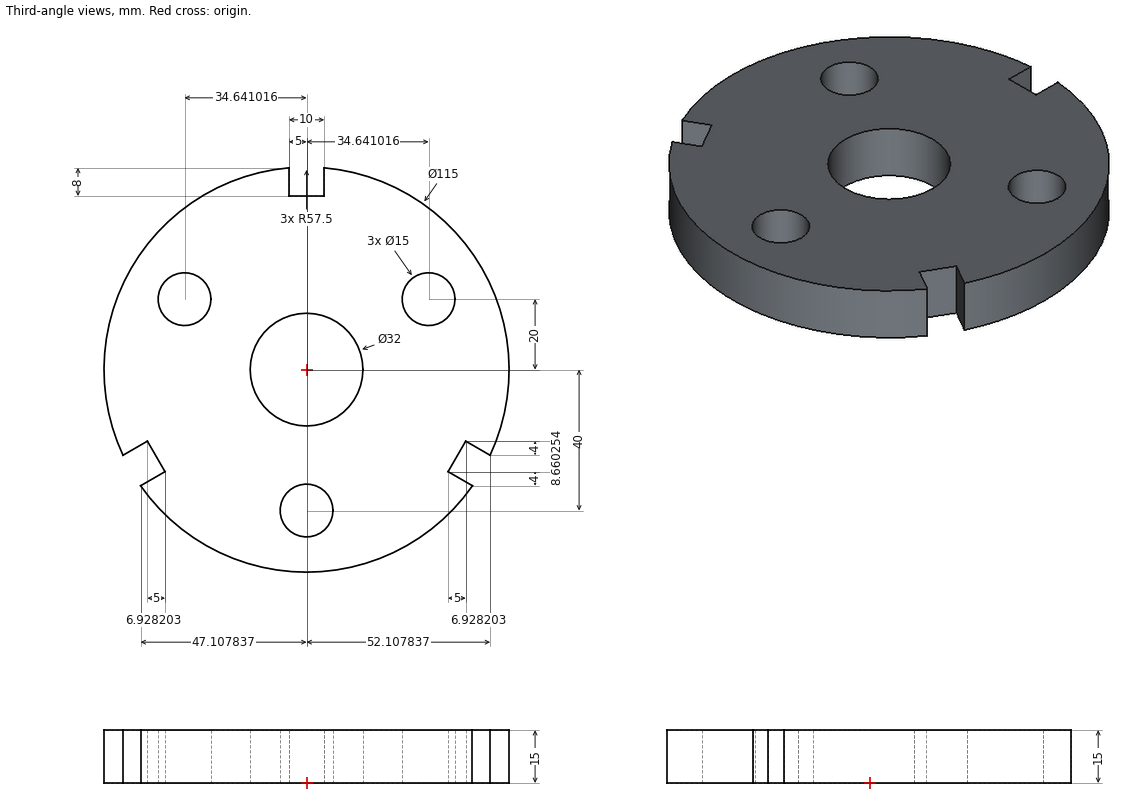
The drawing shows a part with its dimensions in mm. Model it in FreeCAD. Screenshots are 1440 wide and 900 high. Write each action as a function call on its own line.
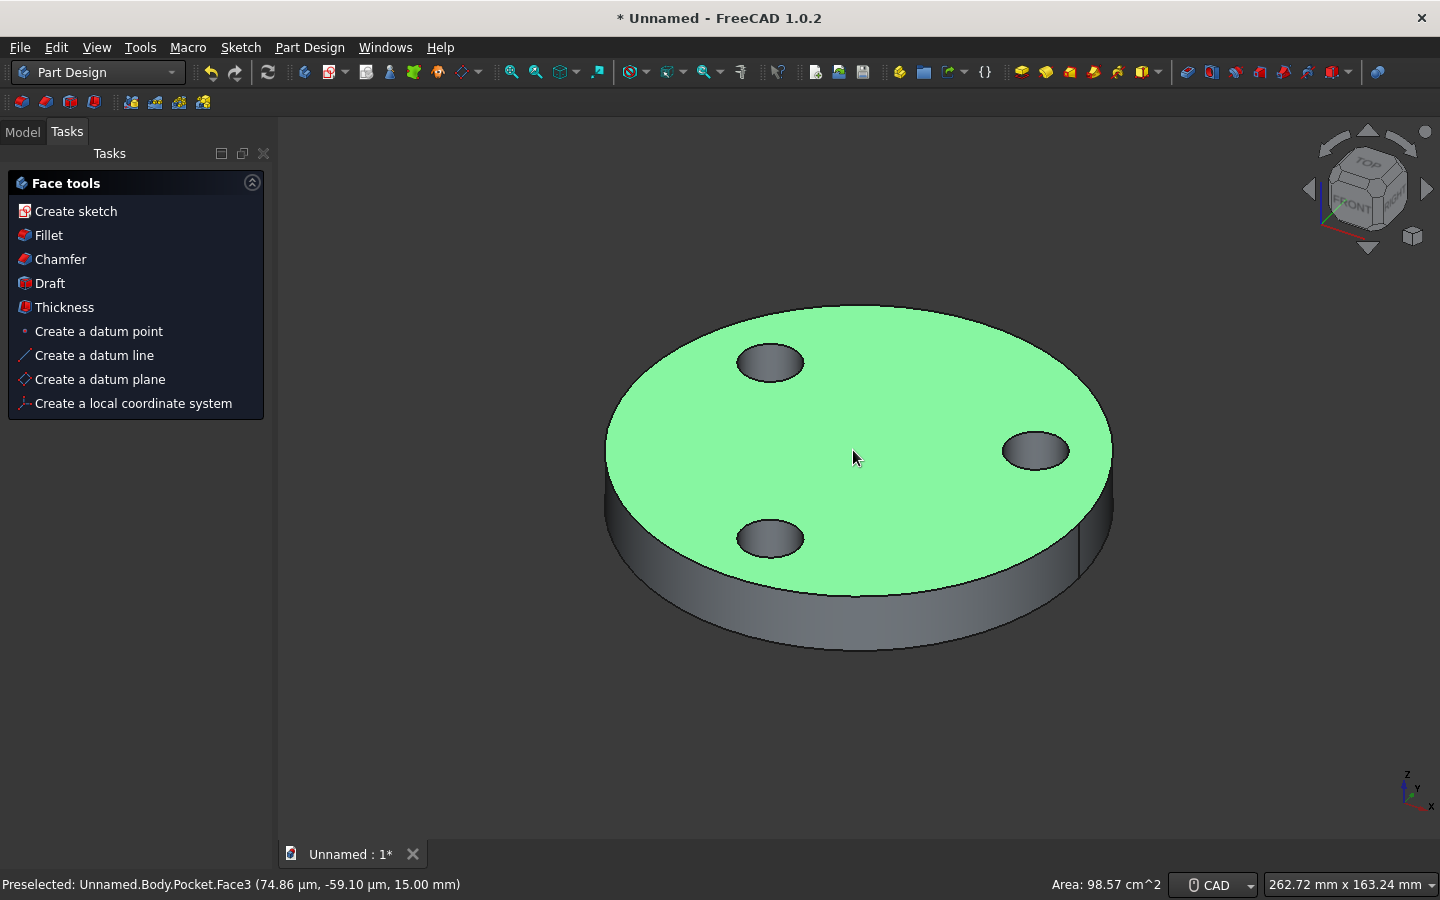
click(330, 72)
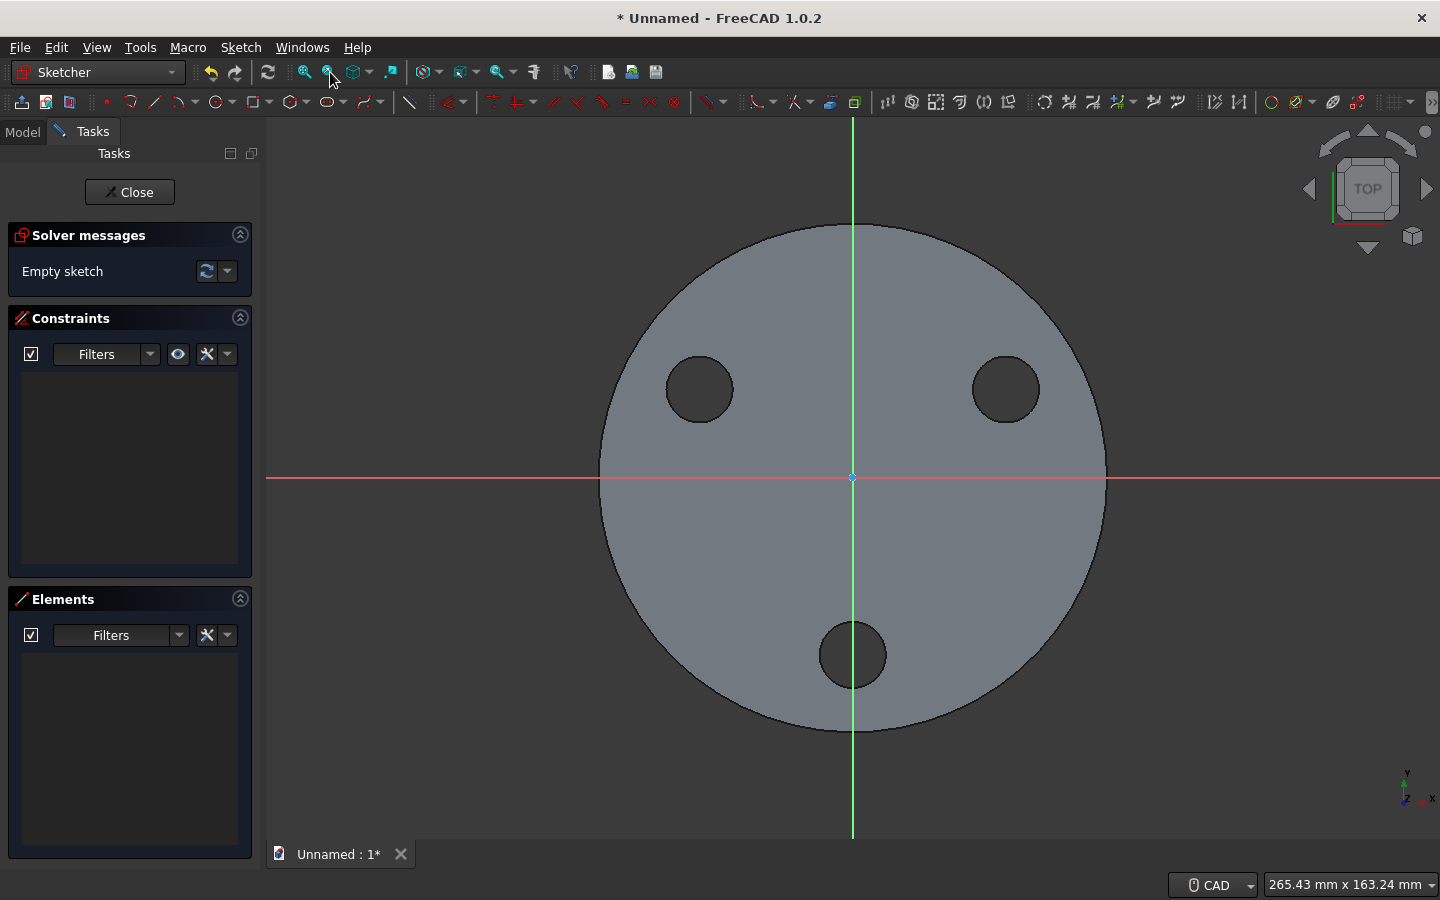
scroll(882, 478, up, 6)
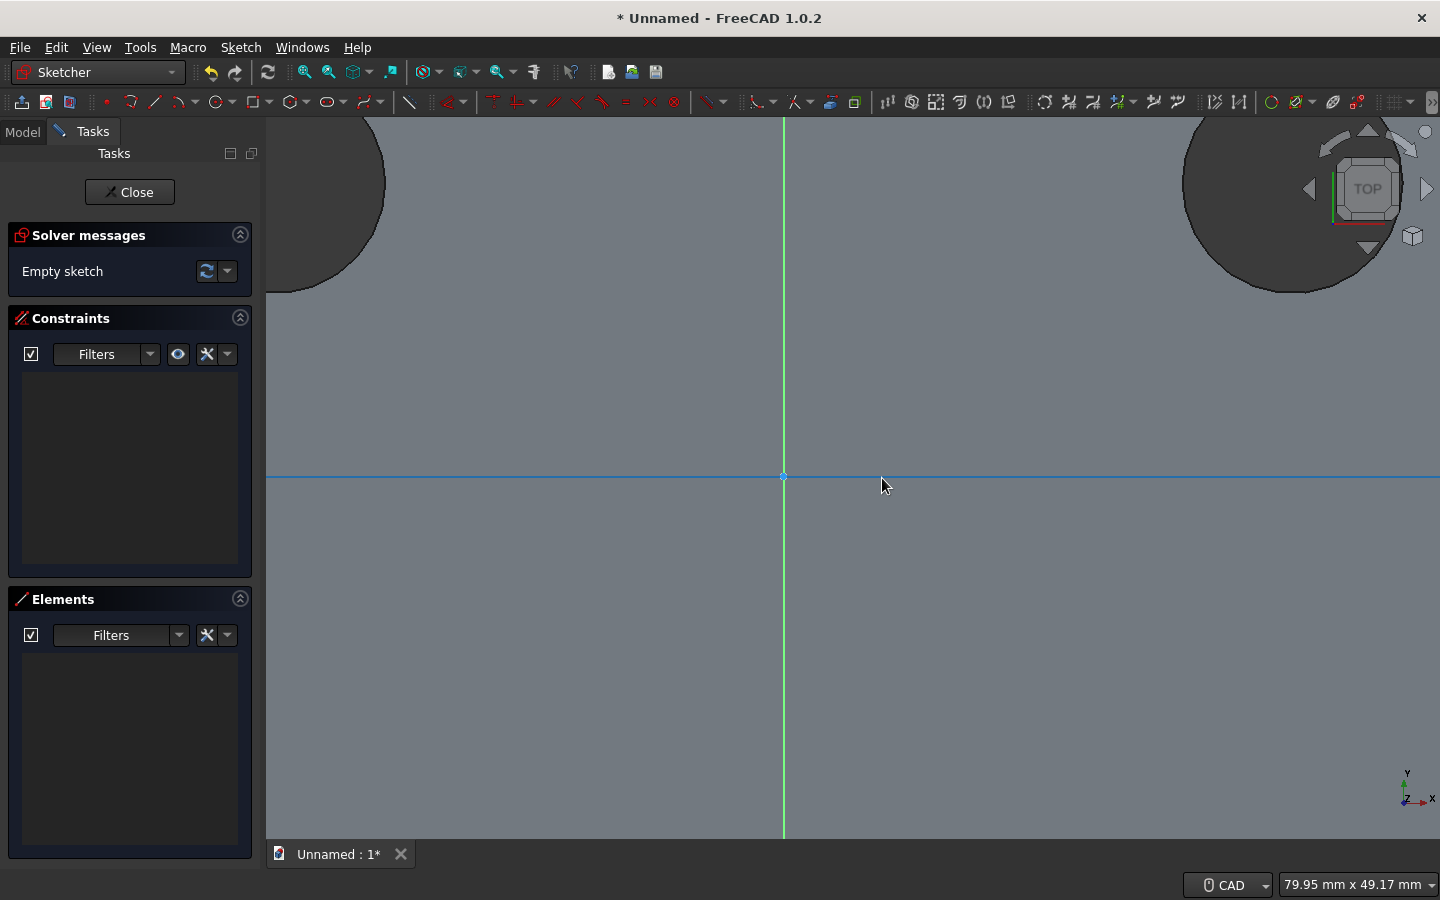
key(g)
key(c)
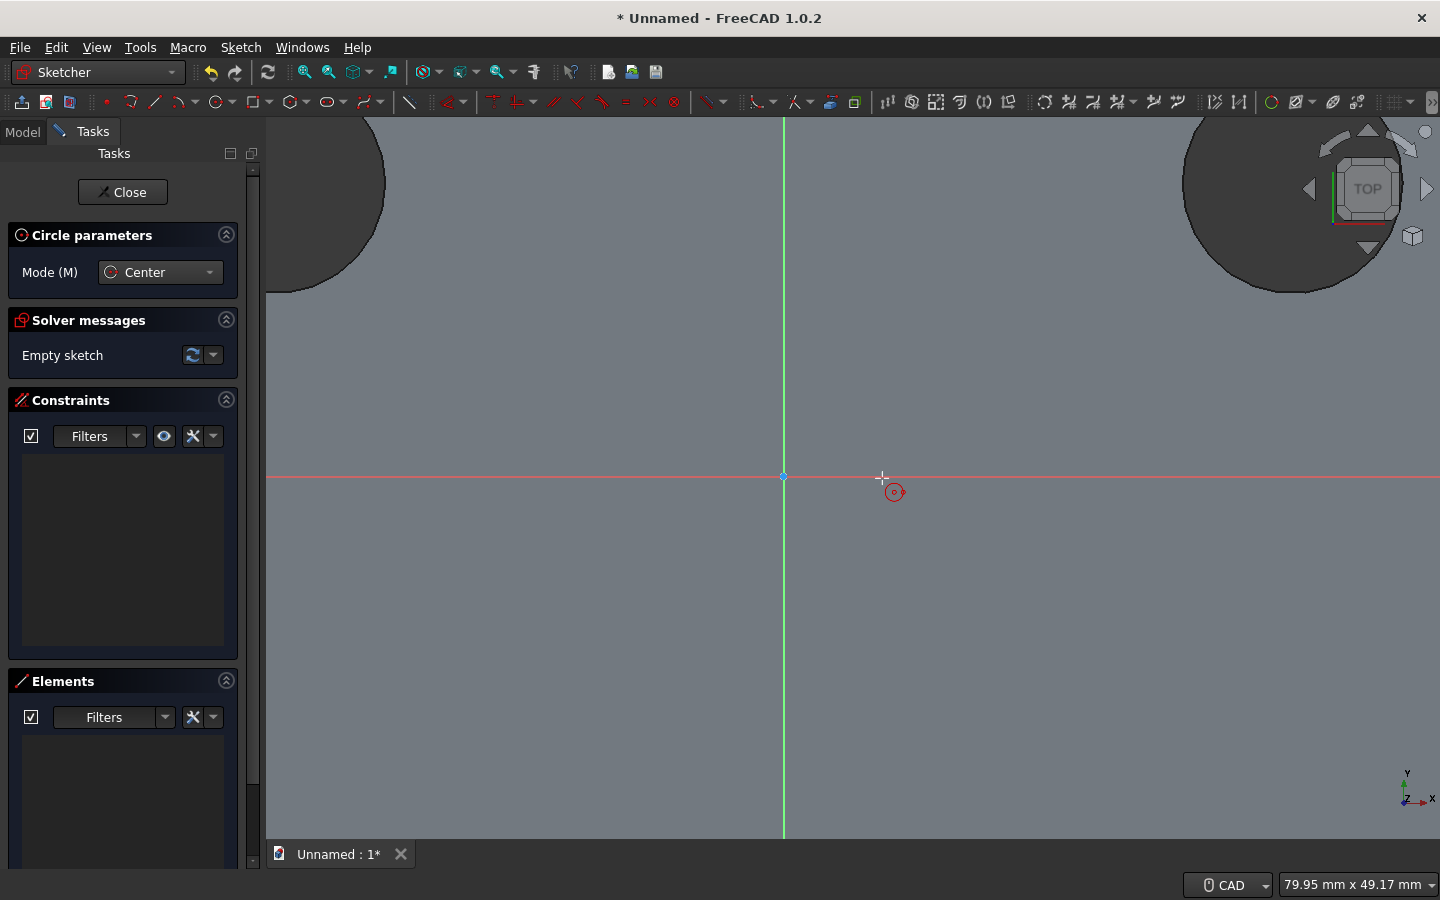
click(784, 477)
move(950, 311)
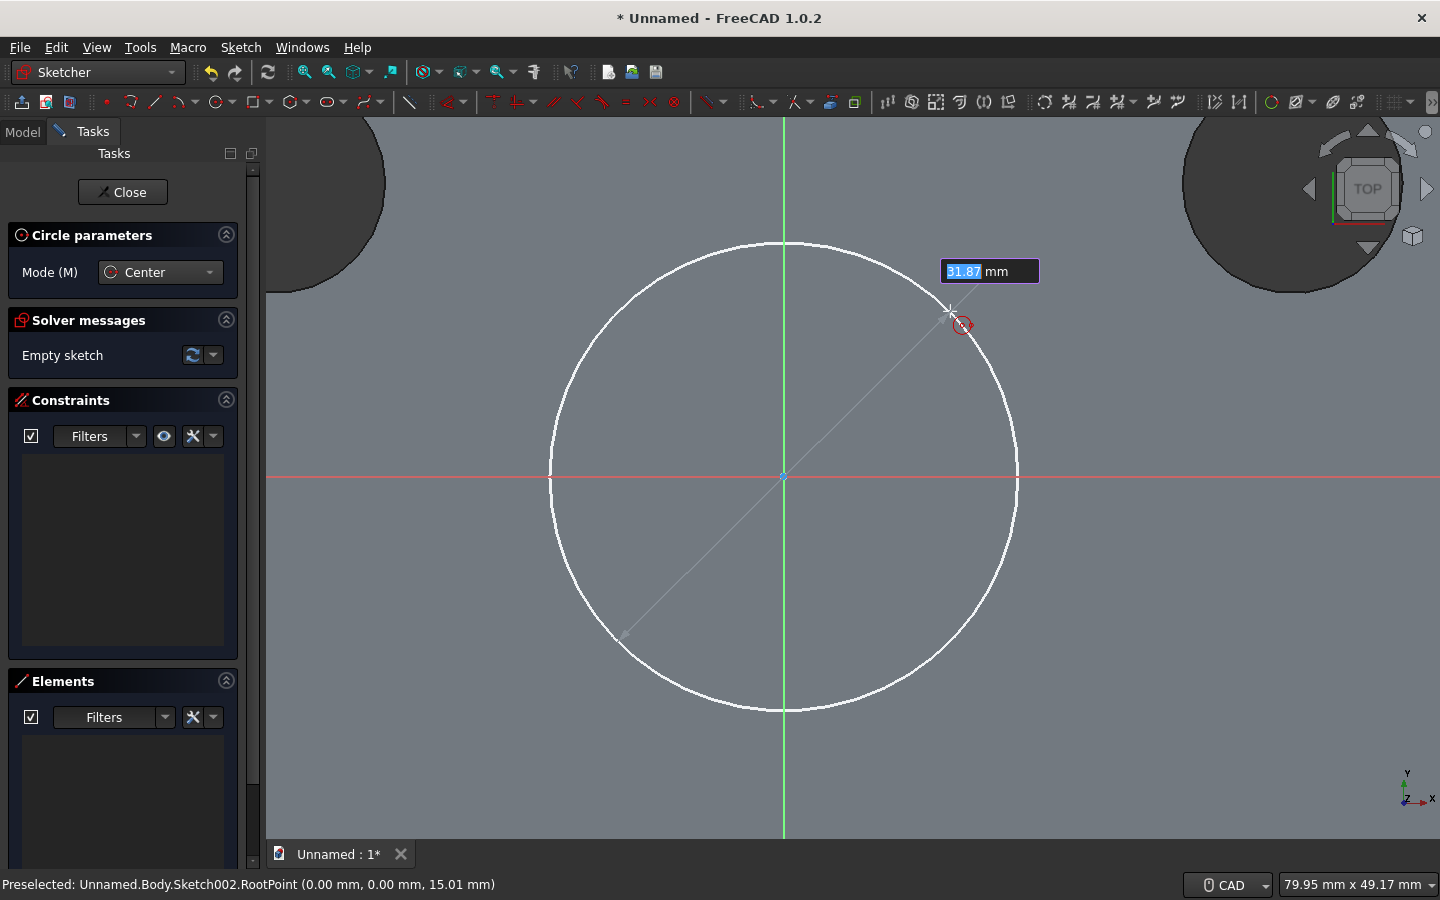
text(32)
key(Return)
key(Escape)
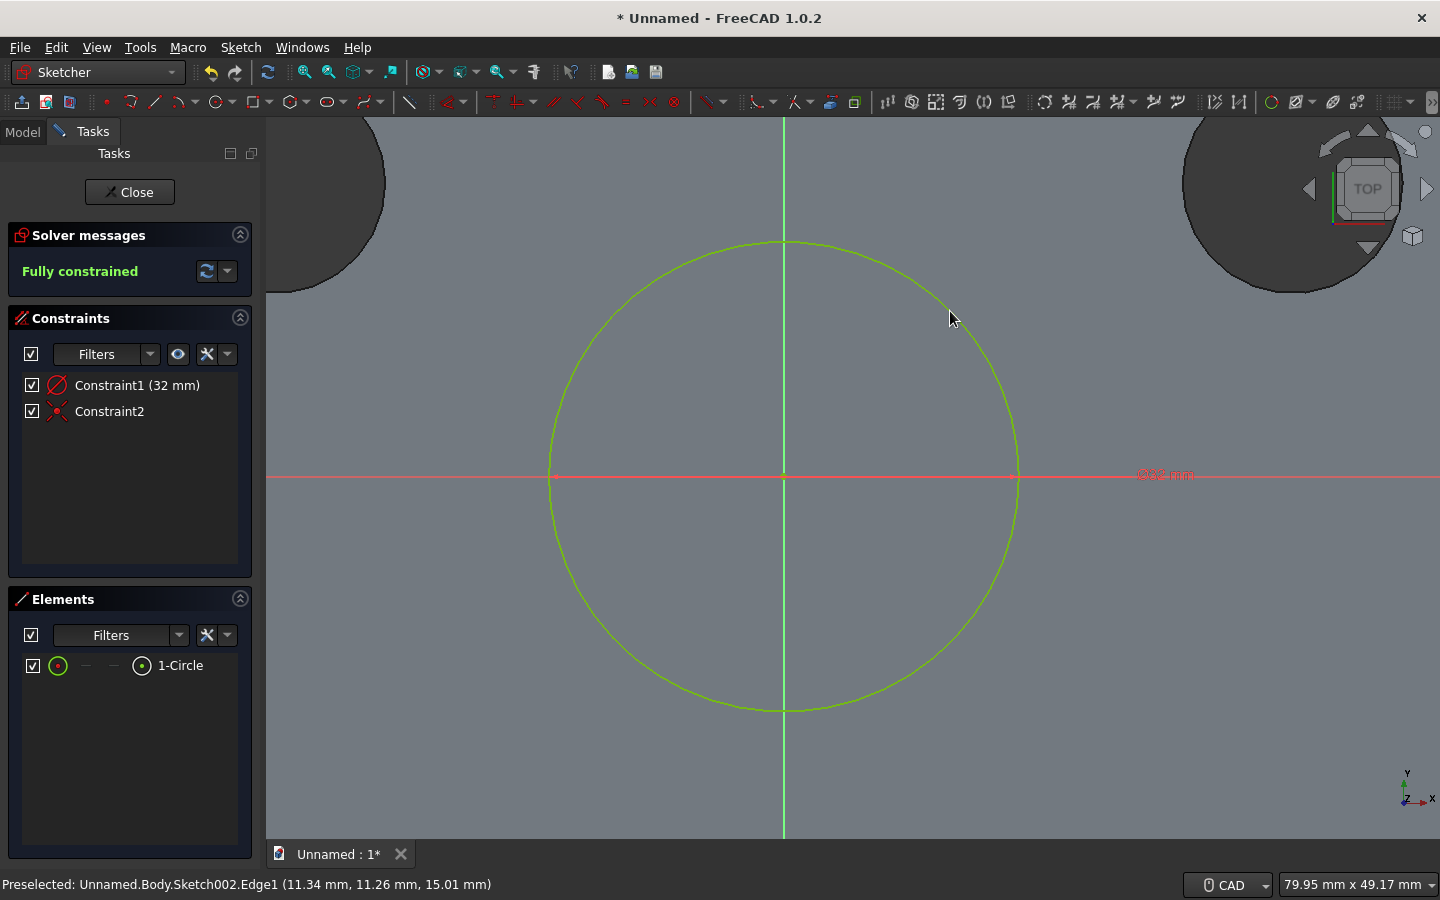
click(130, 192)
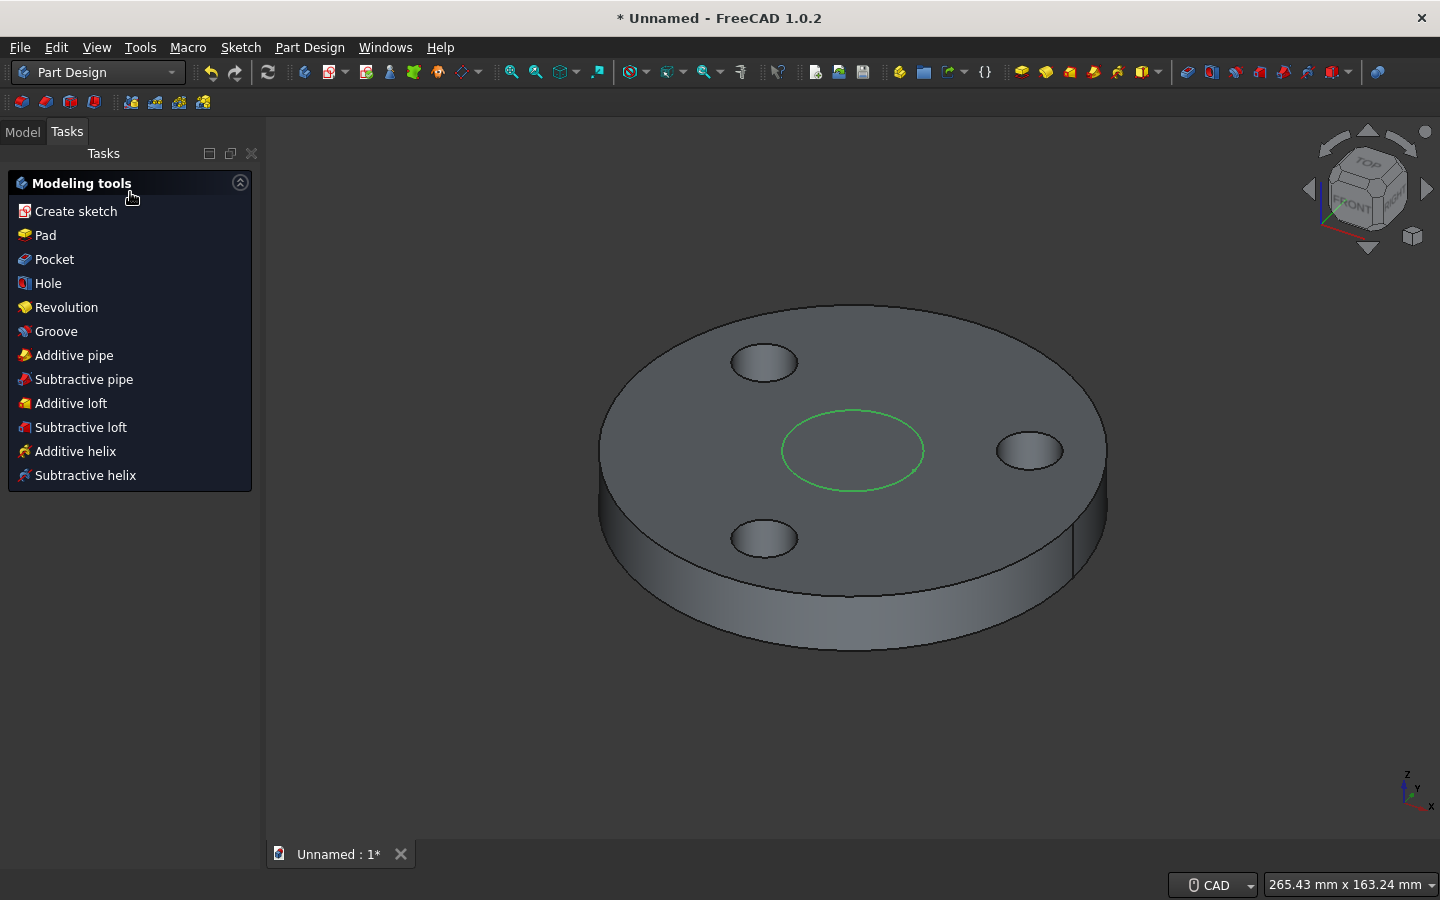
click(1188, 72)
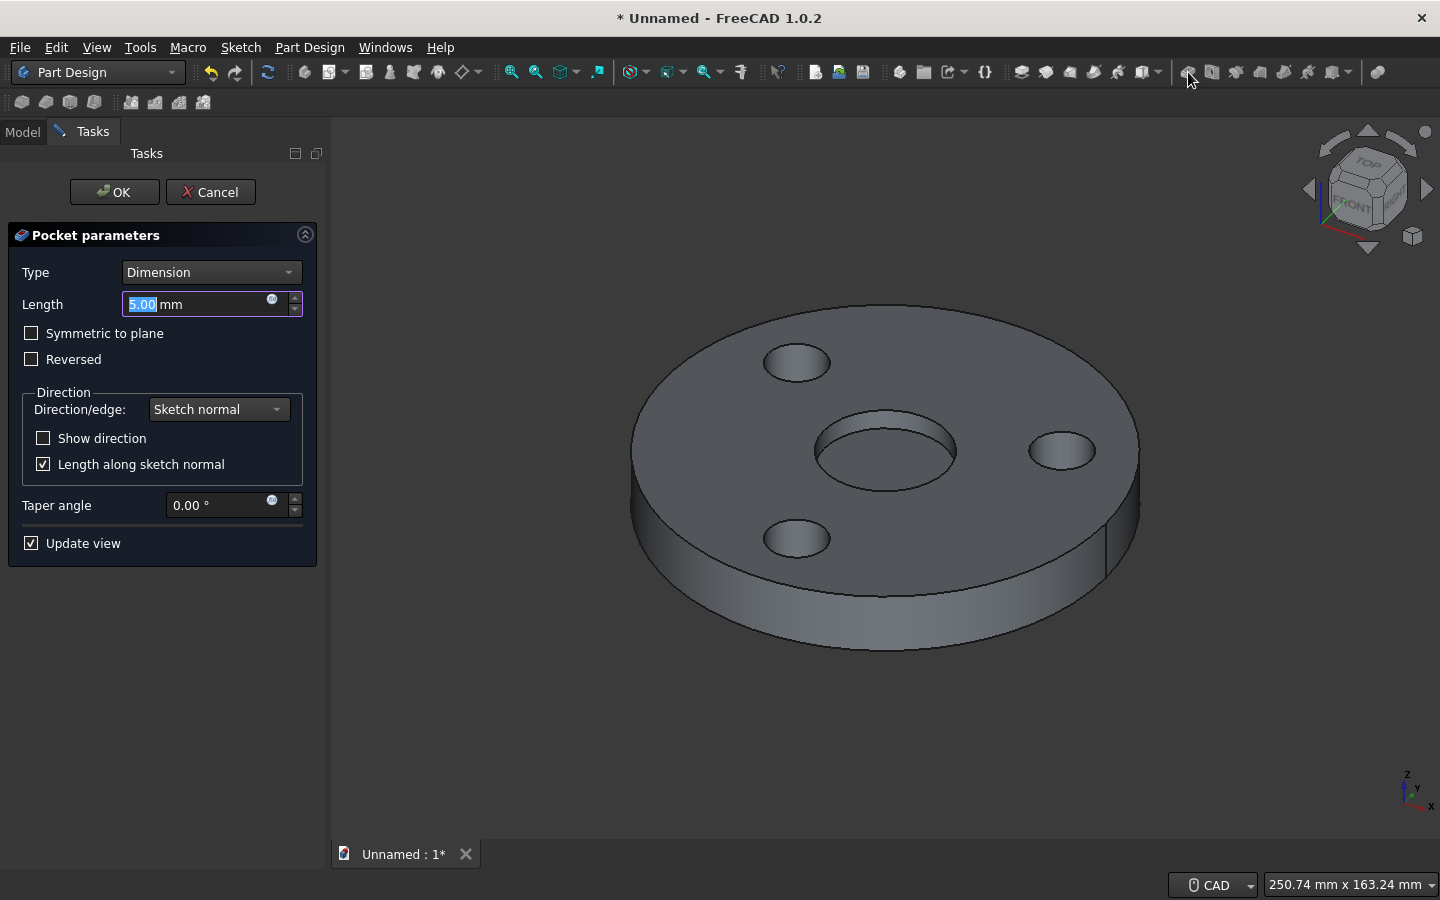
text(15)
key(Tab)